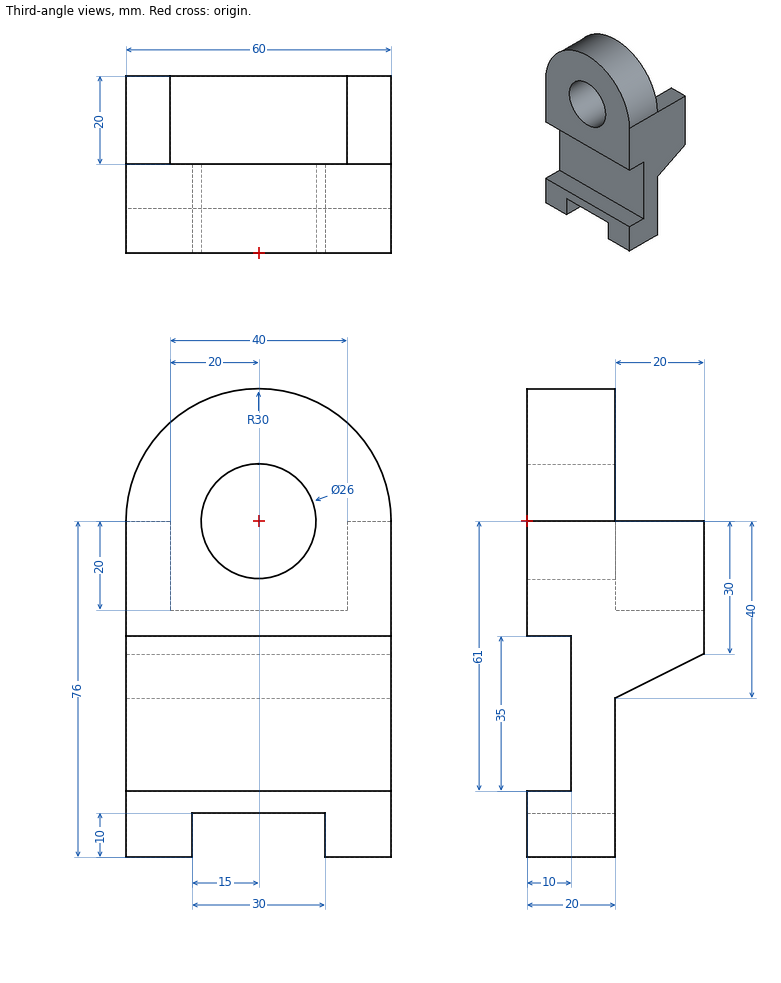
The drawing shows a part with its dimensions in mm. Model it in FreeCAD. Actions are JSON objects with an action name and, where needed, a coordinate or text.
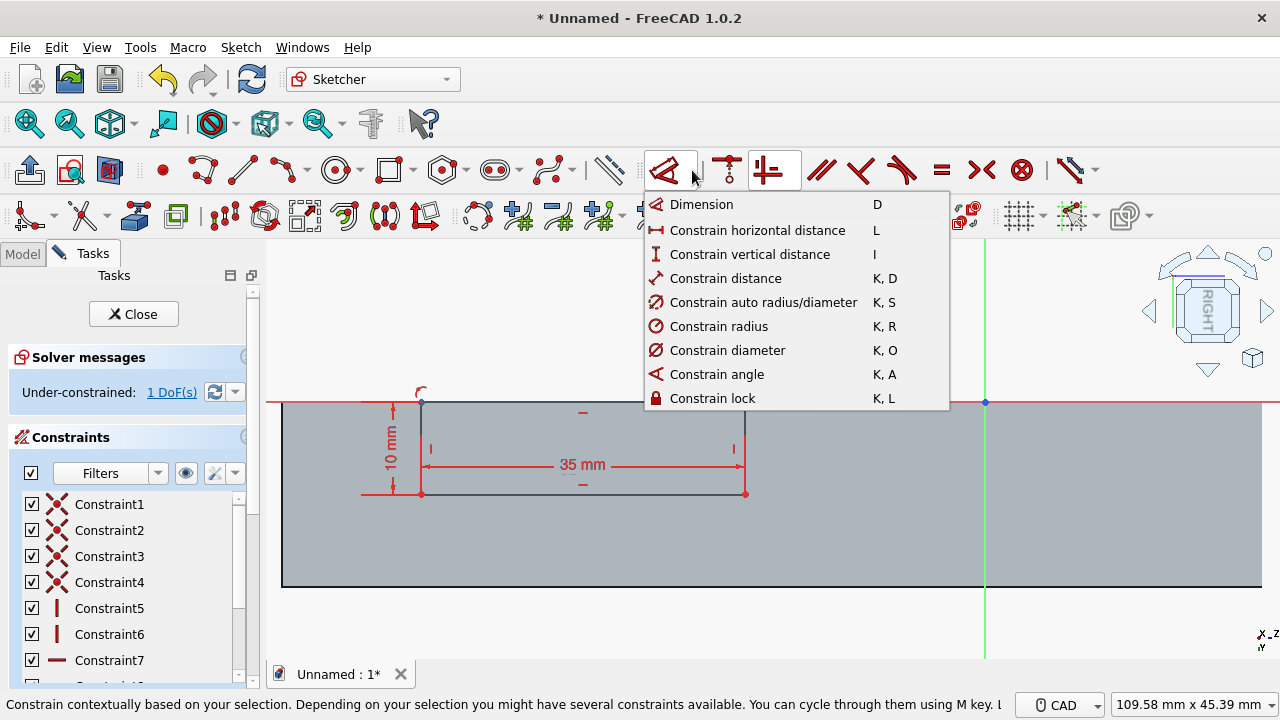
{"action": "left_click", "coordinate": [797, 230]}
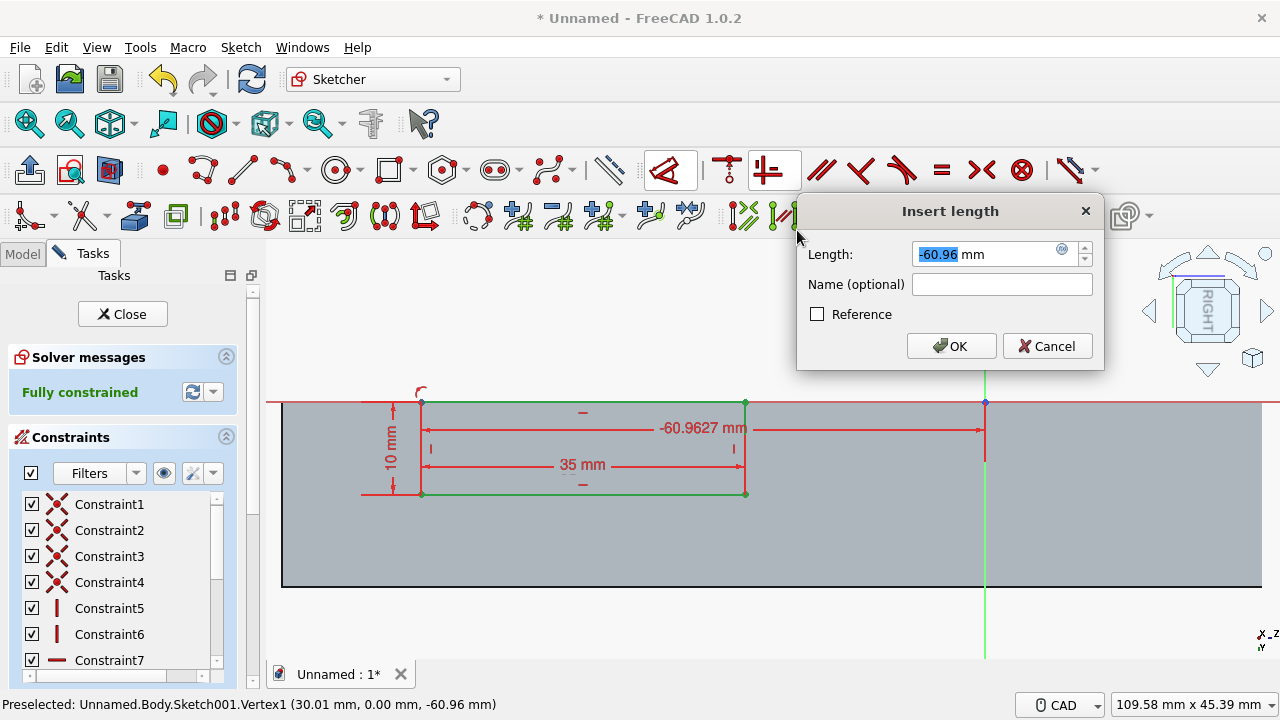
{"action": "type", "text": "-61"}
{"action": "key", "text": "Return"}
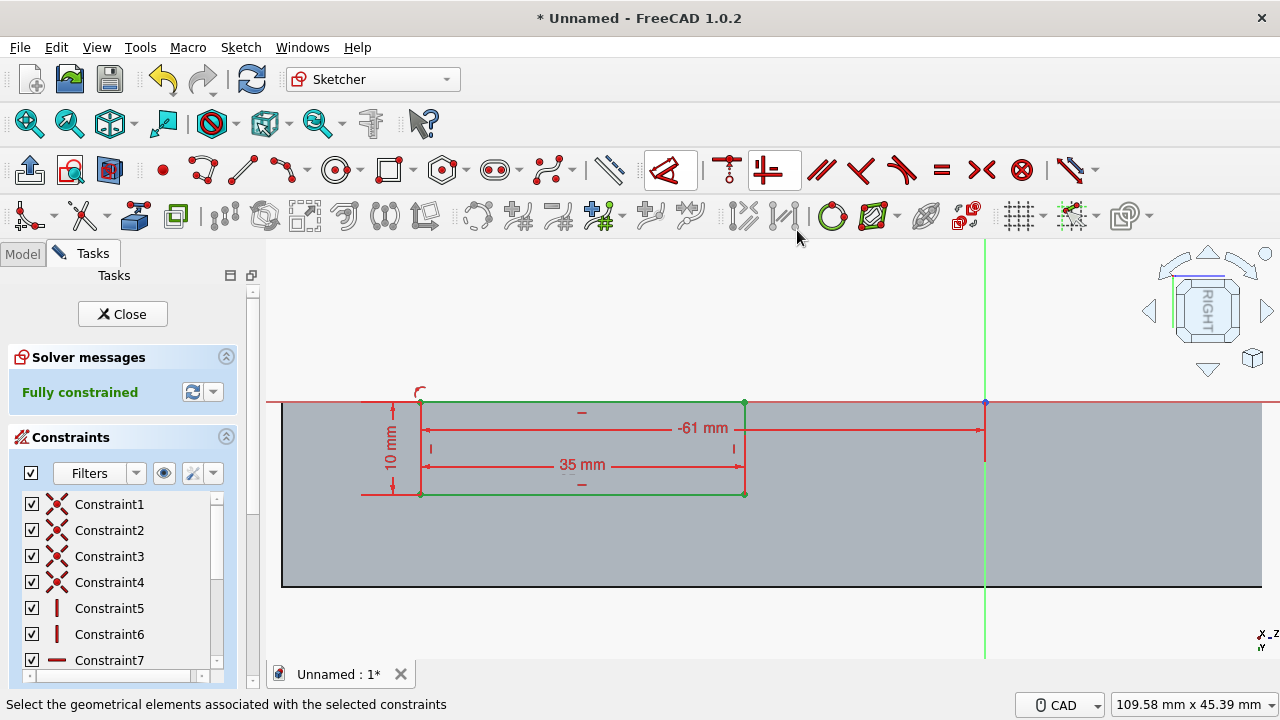
{"action": "left_click", "coordinate": [123, 314]}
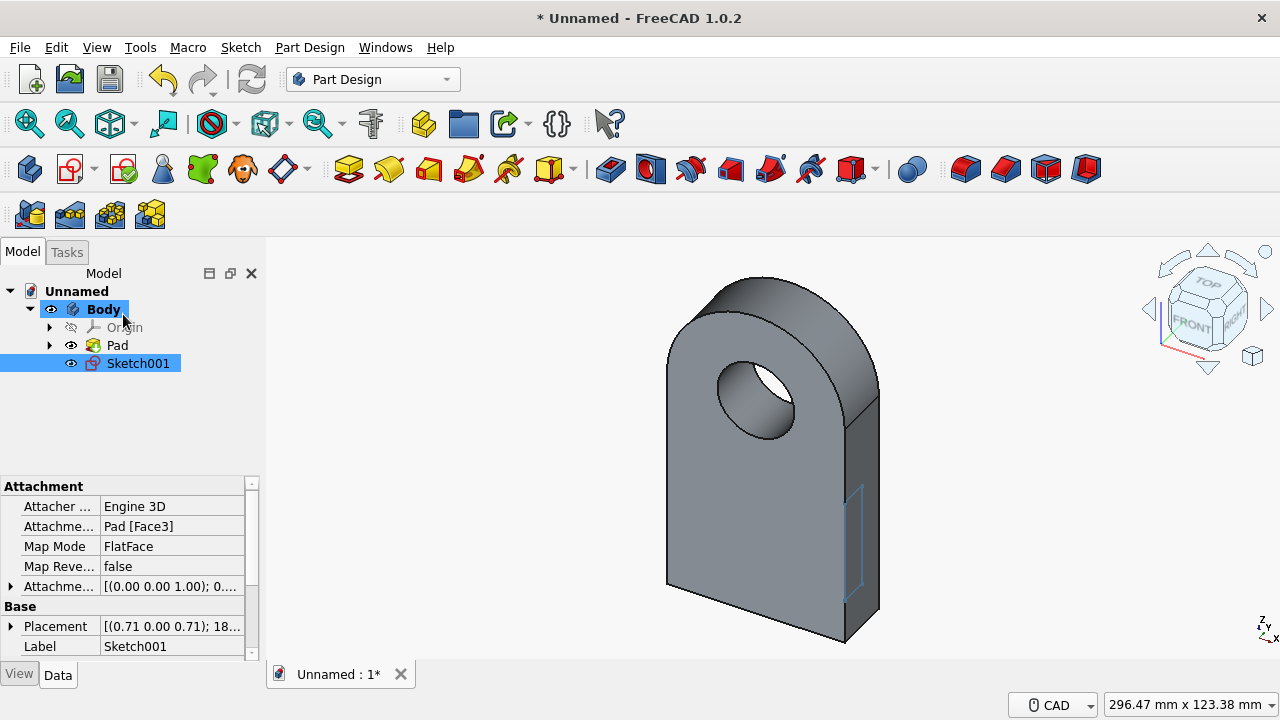
{"action": "left_click", "coordinate": [612, 170]}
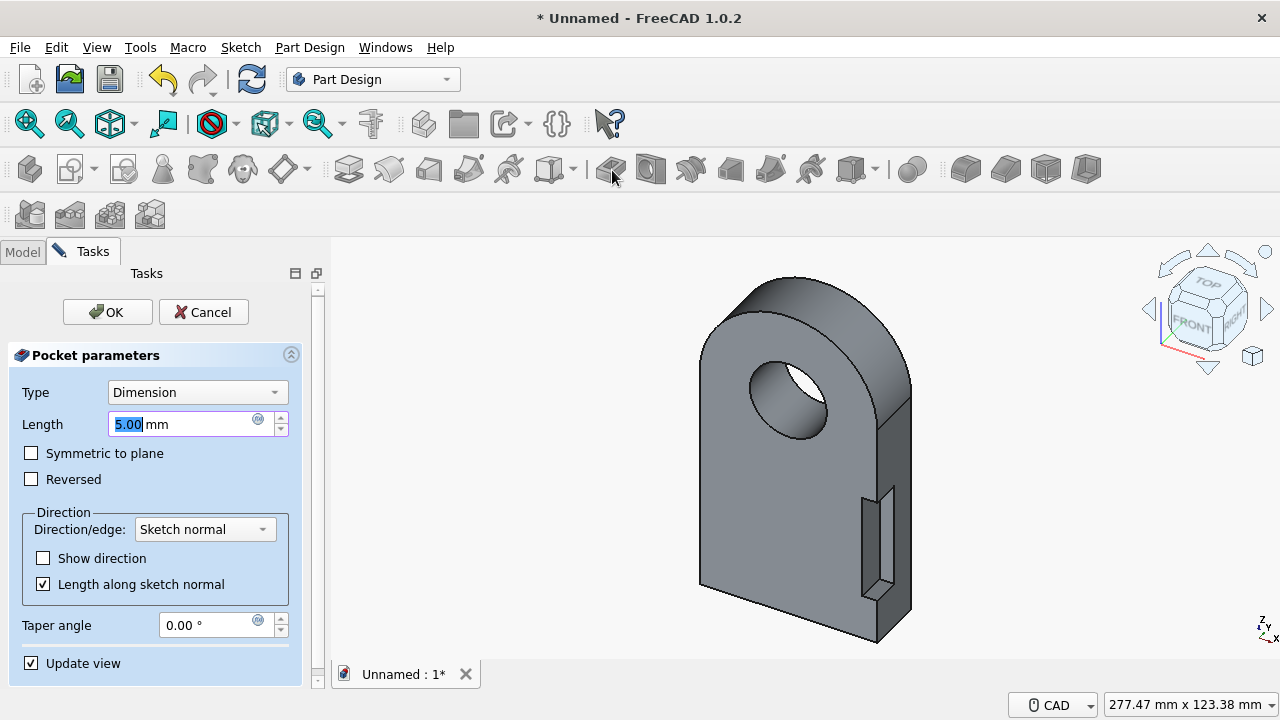
{"action": "left_click", "coordinate": [198, 392]}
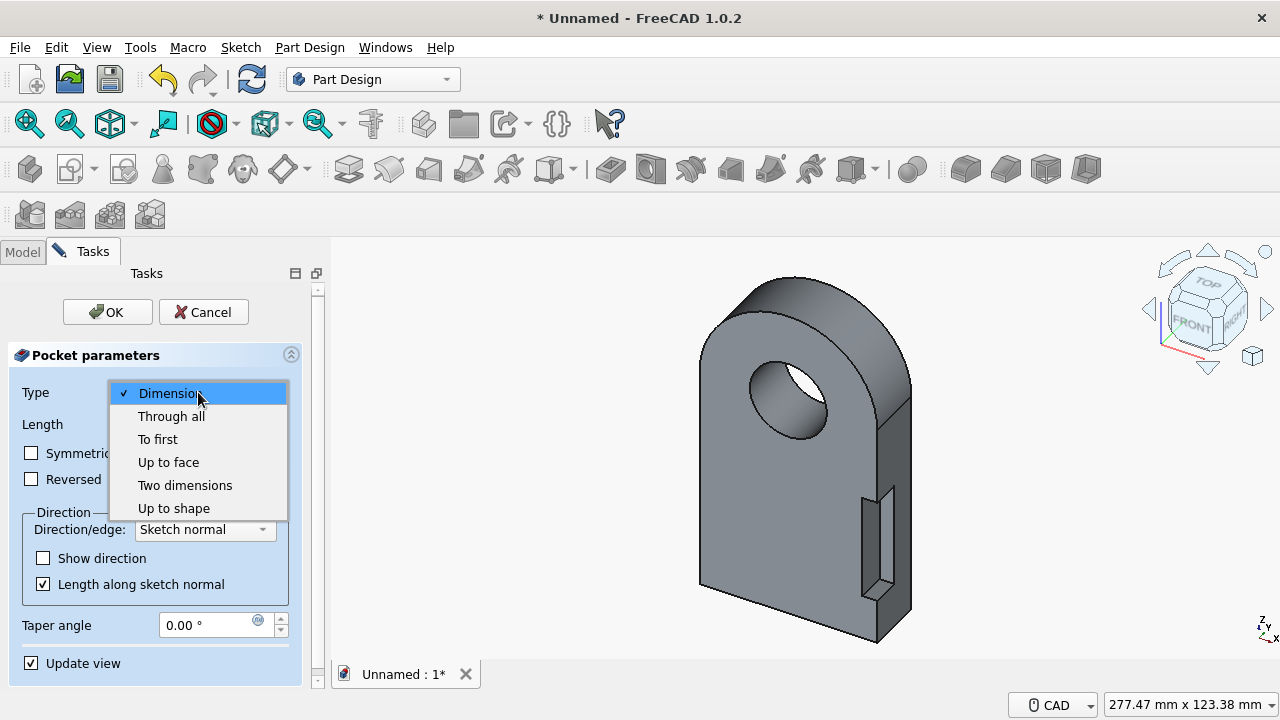
{"action": "left_click", "coordinate": [198, 440]}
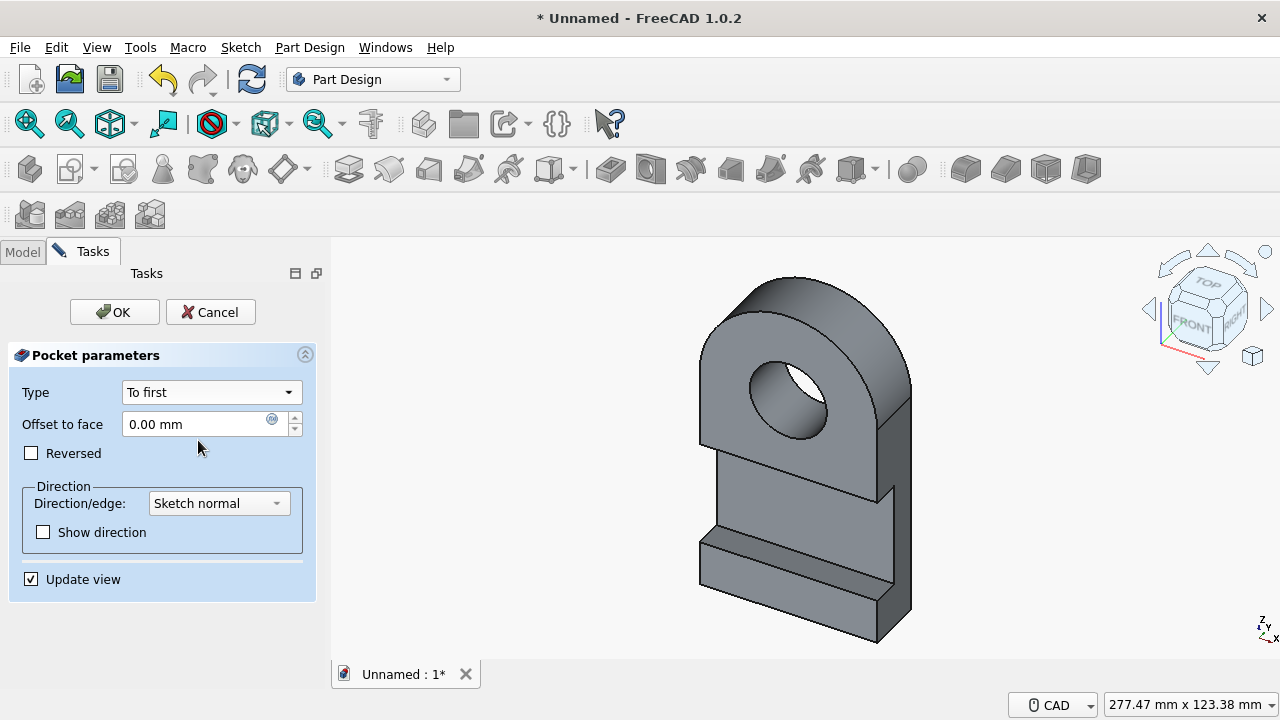
{"action": "left_click", "coordinate": [115, 312]}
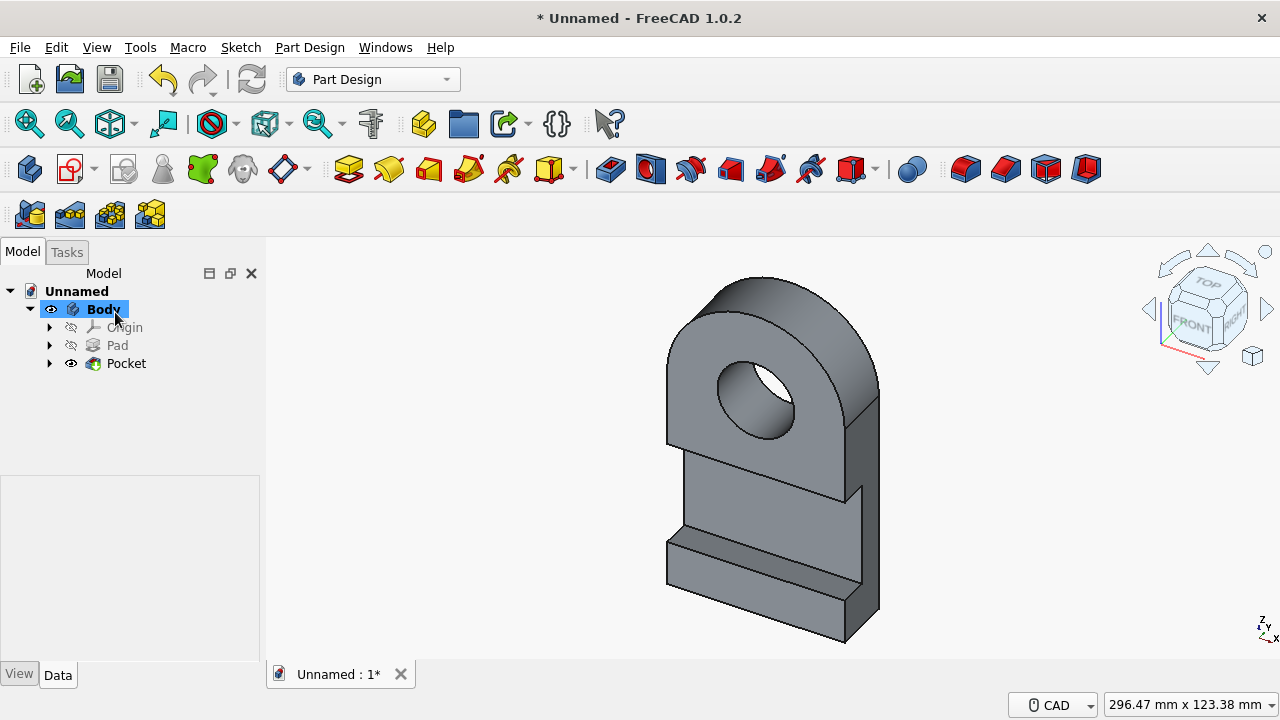
{"action": "key", "text": "4"}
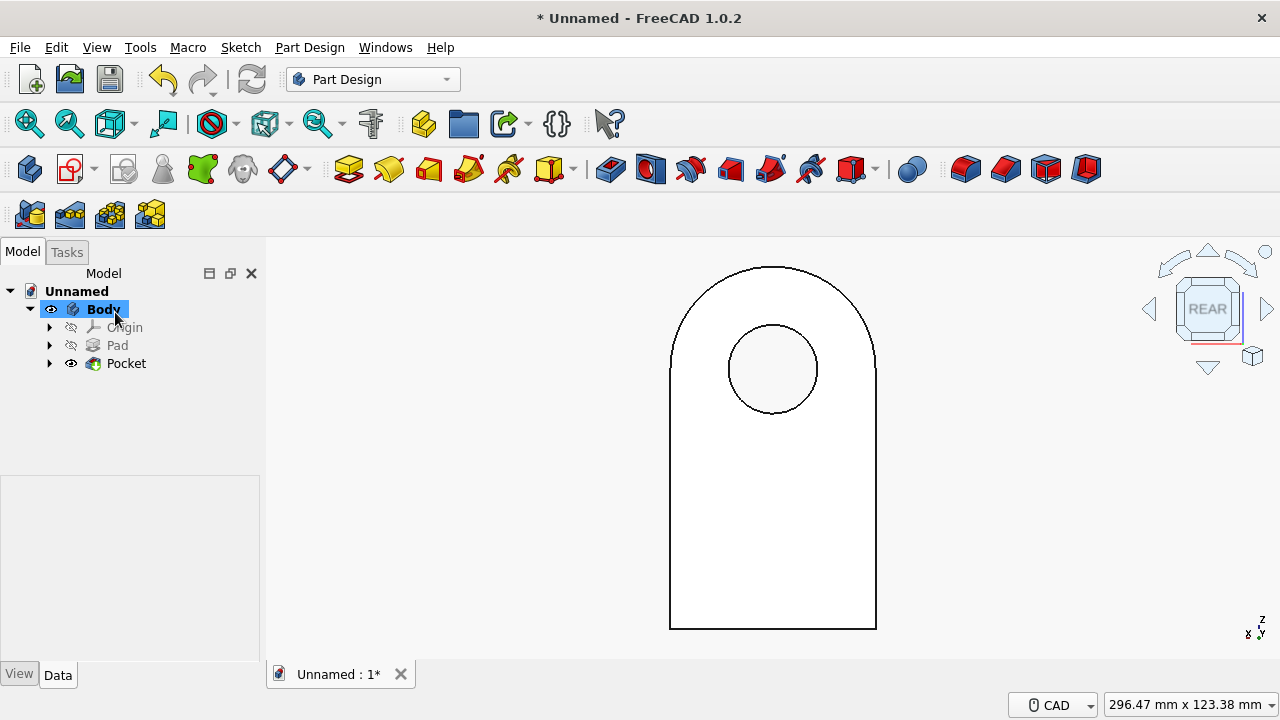
{"action": "left_click", "coordinate": [773, 499]}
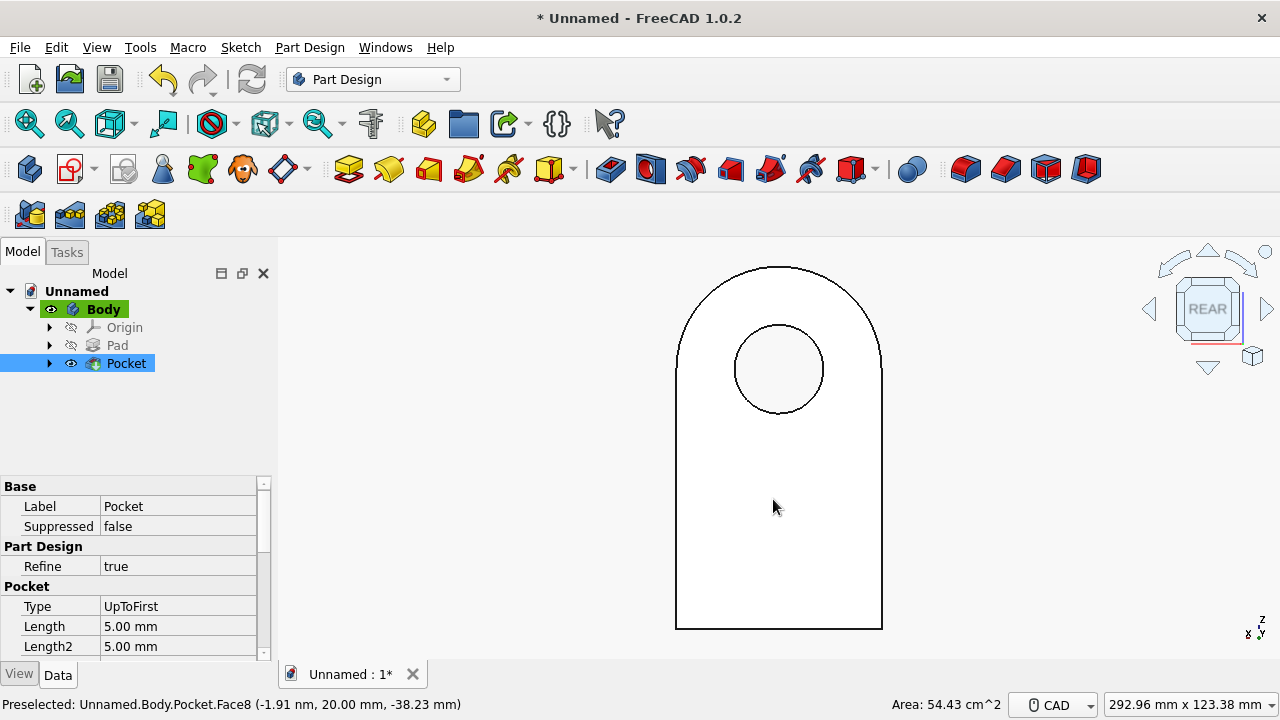
{"action": "left_click", "coordinate": [70, 170]}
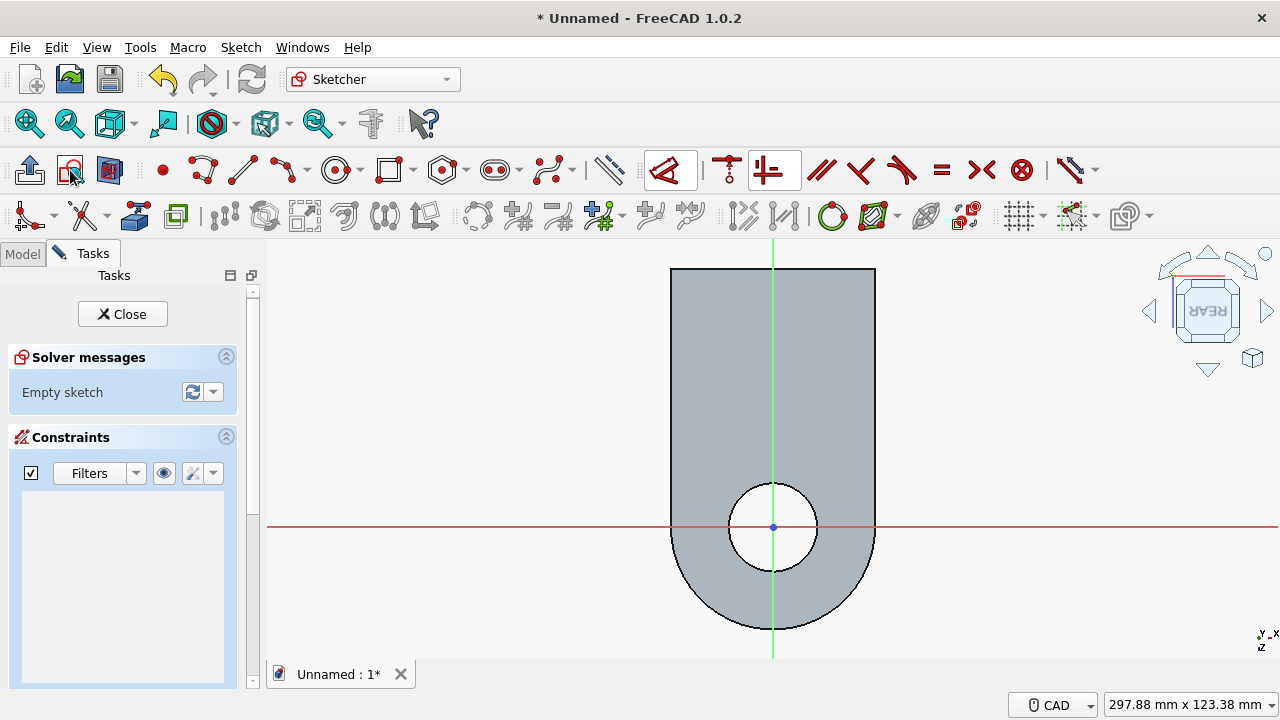
{"action": "scroll", "coordinate": [704, 449], "scroll_direction": "down", "scroll_amount": 5}